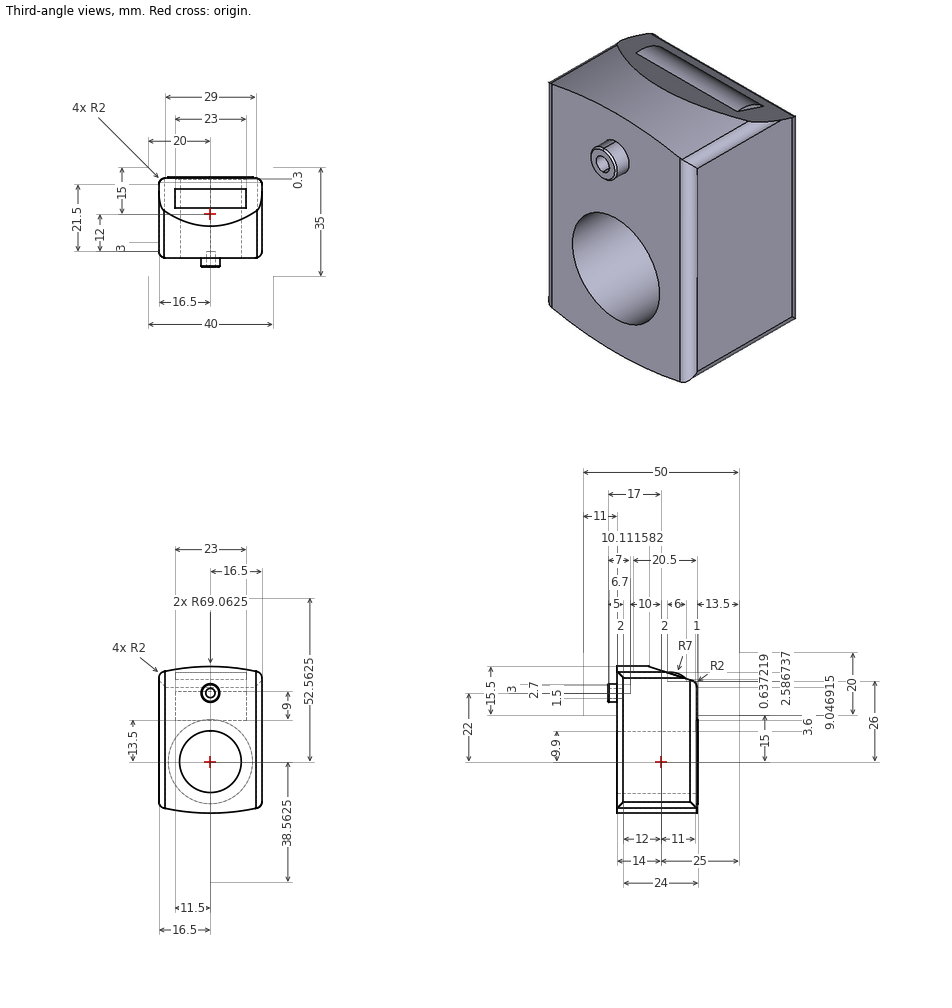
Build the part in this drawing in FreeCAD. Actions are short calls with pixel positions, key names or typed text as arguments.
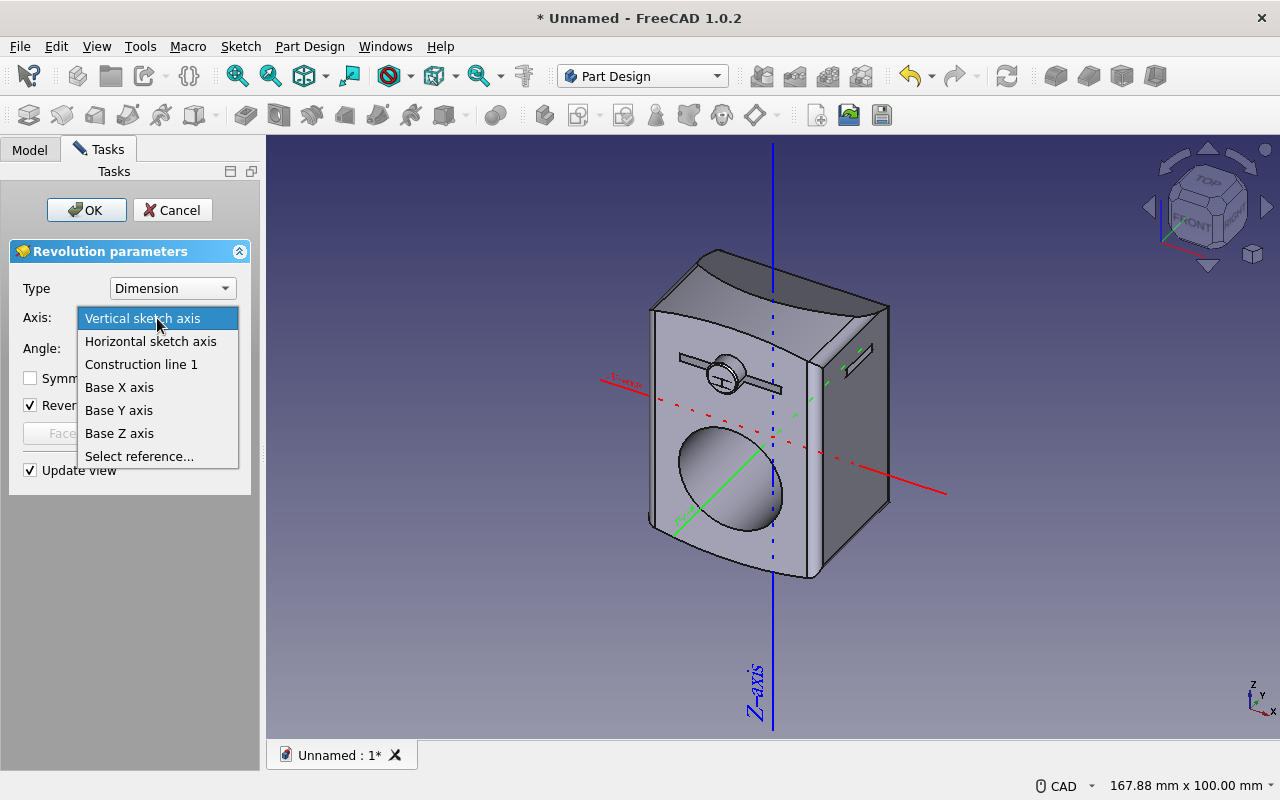
click(156, 364)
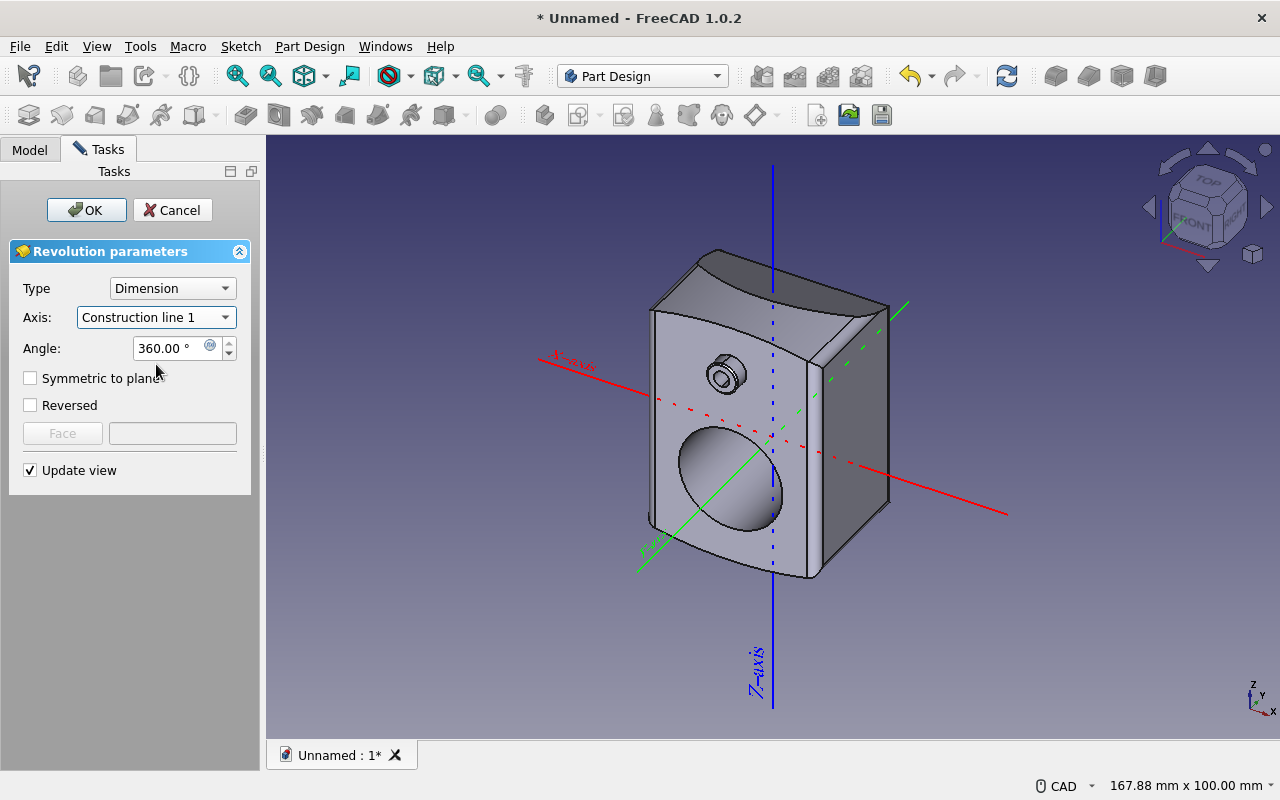
click(87, 210)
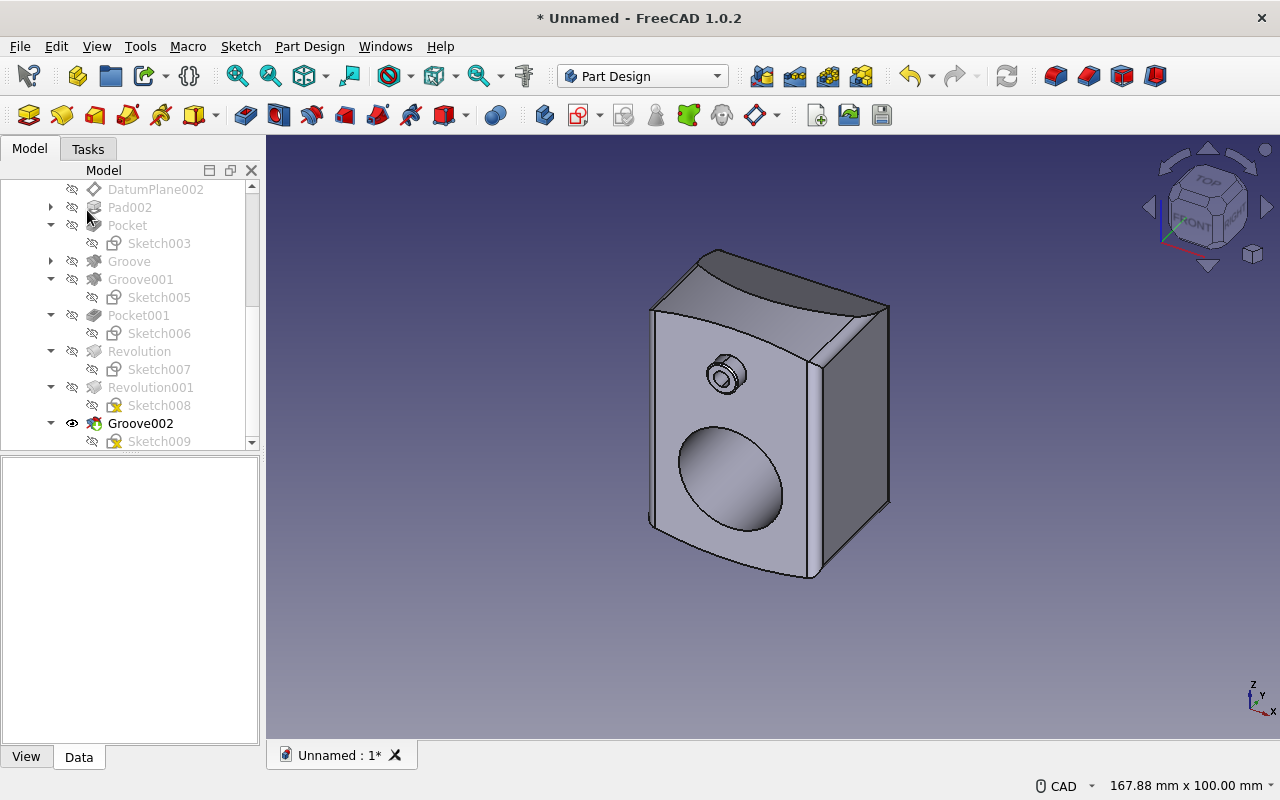
click(578, 116)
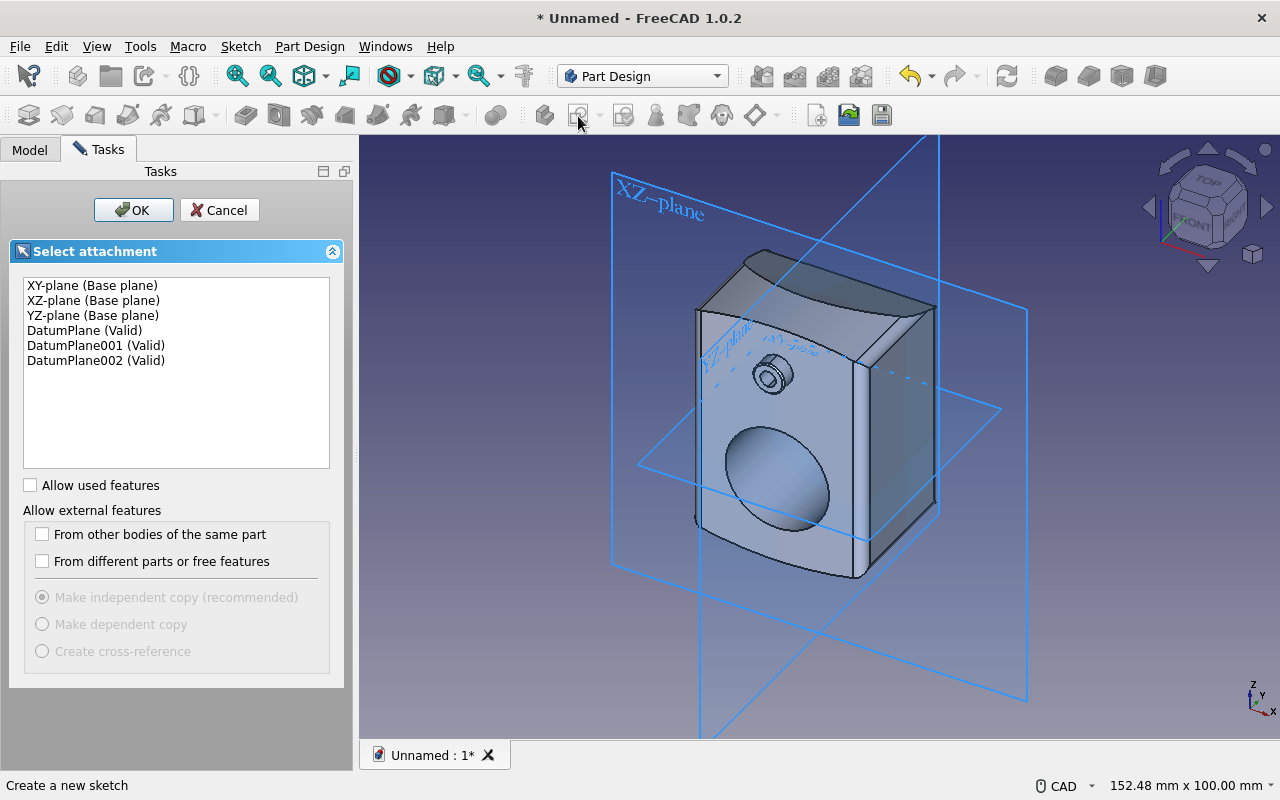
click(84, 316)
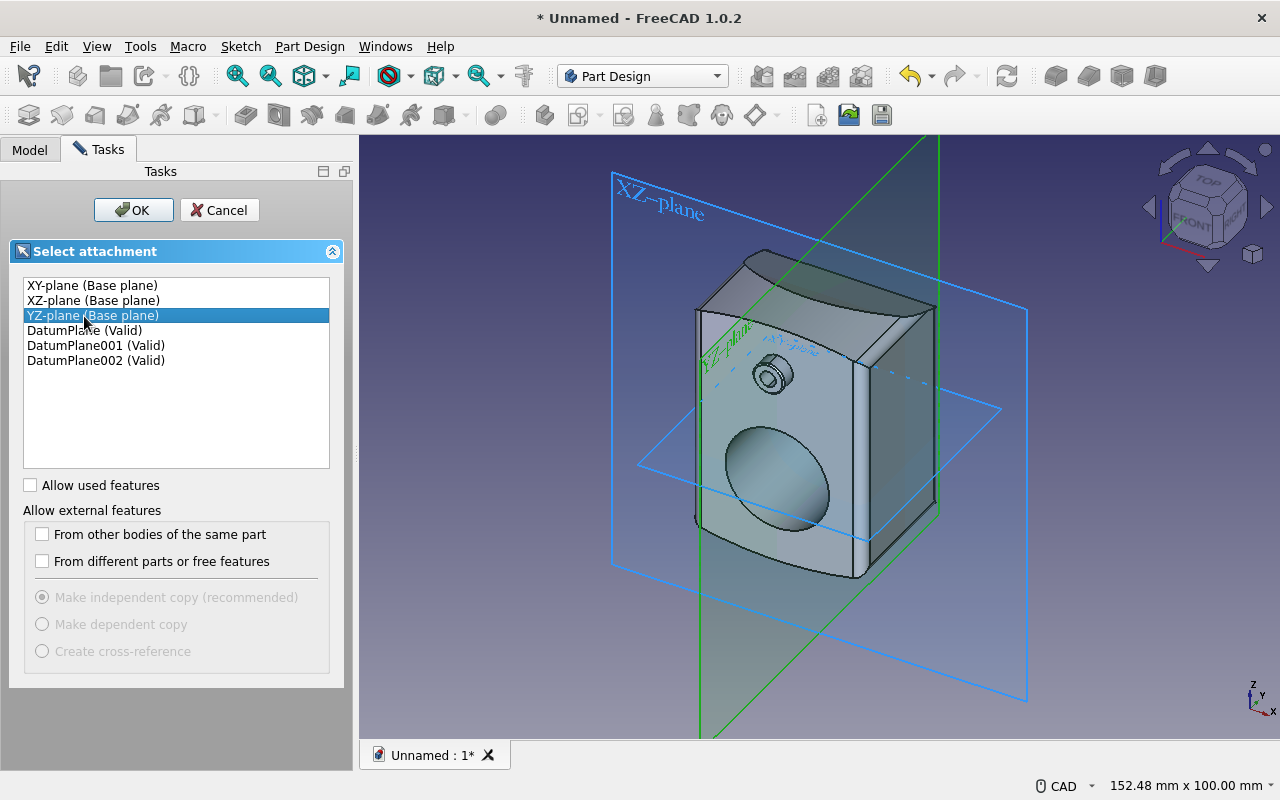
click(134, 210)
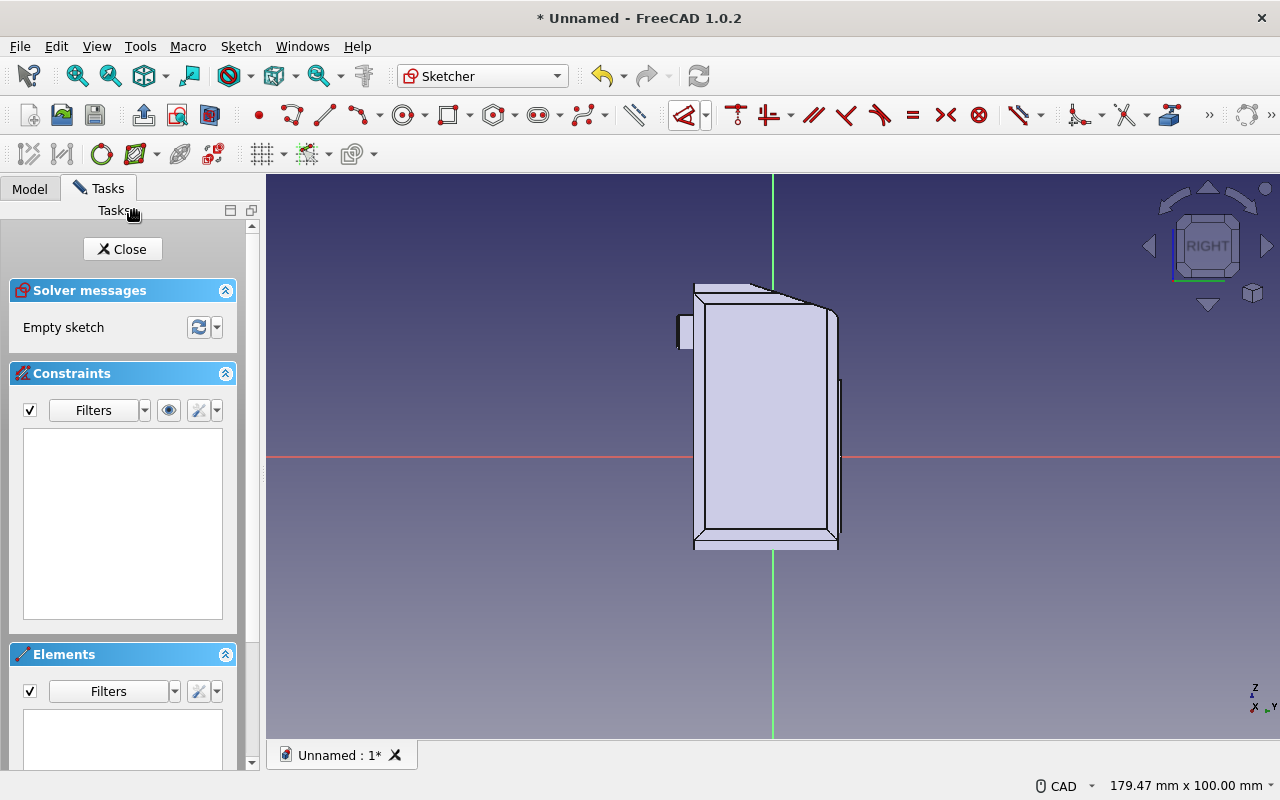
click(210, 116)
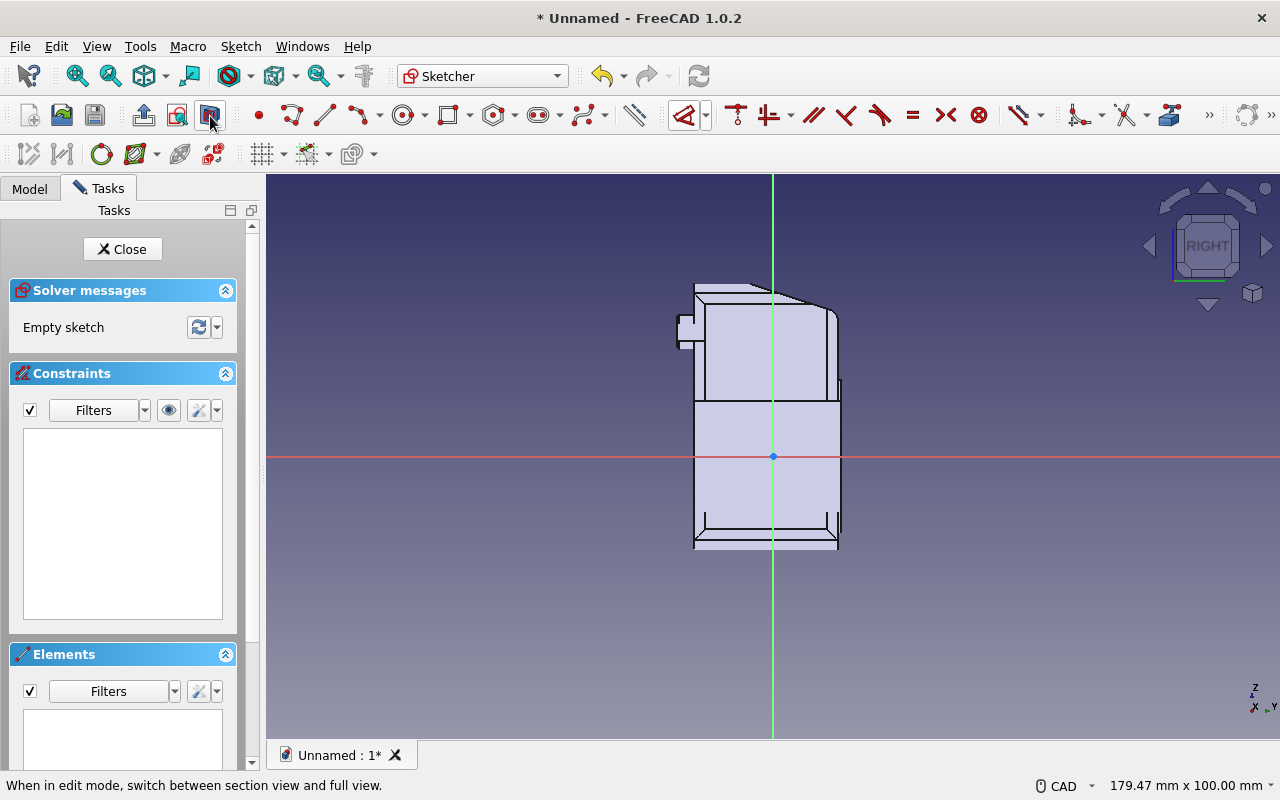
scroll(808, 292, up, 14)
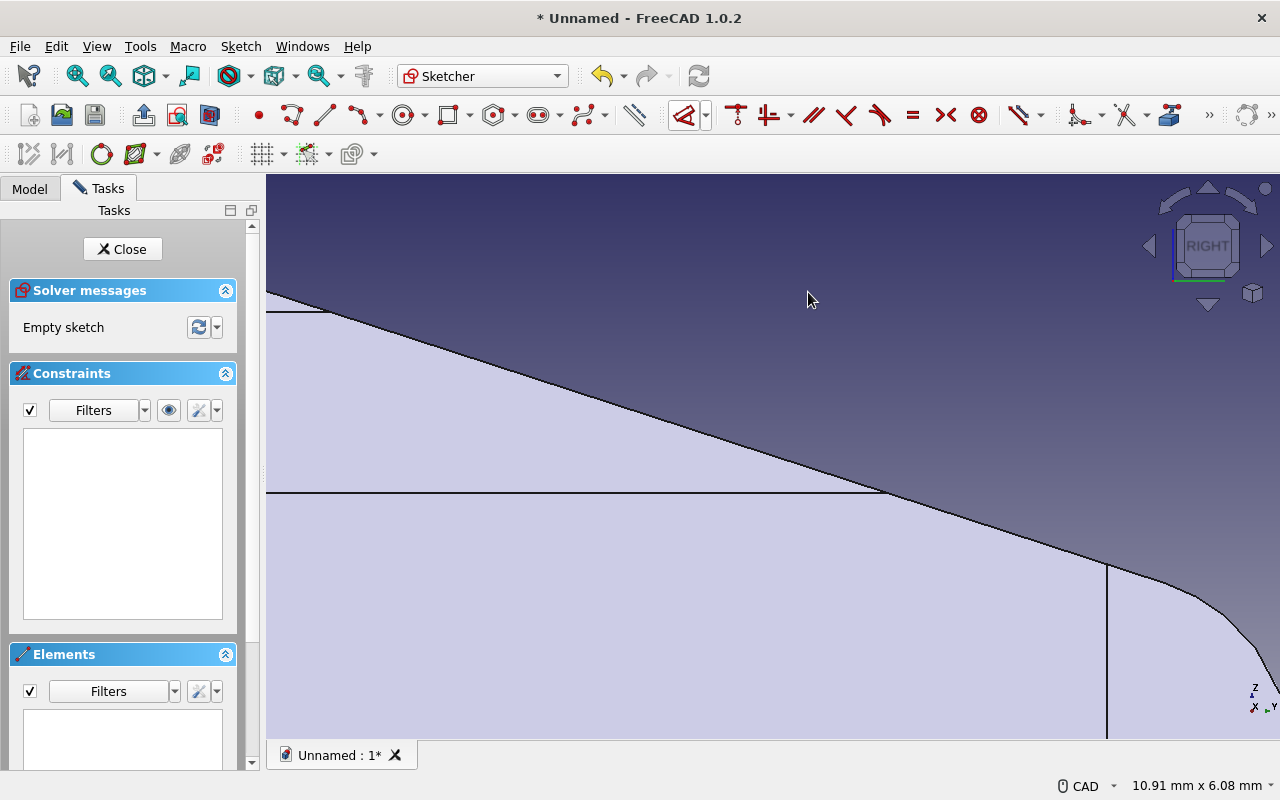
click(292, 116)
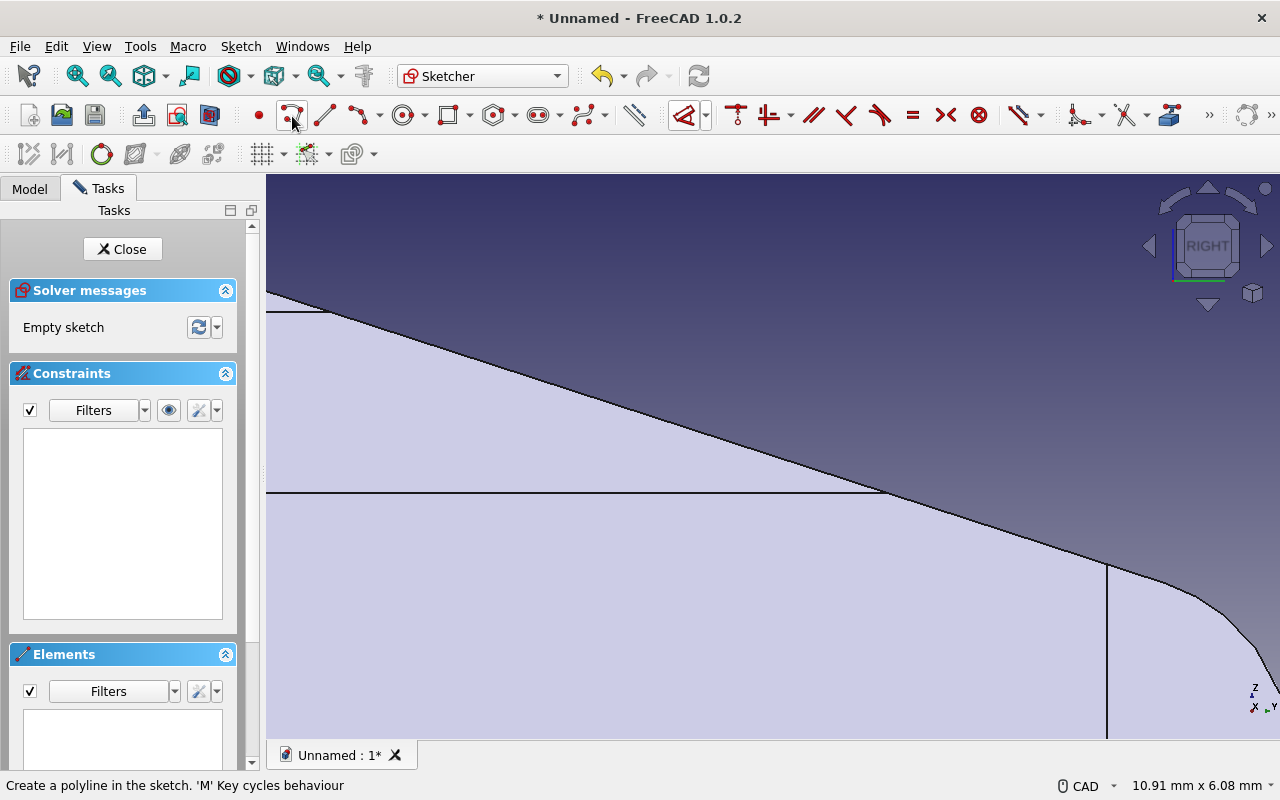
click(410, 338)
click(410, 578)
click(967, 578)
click(967, 519)
right_click(967, 519)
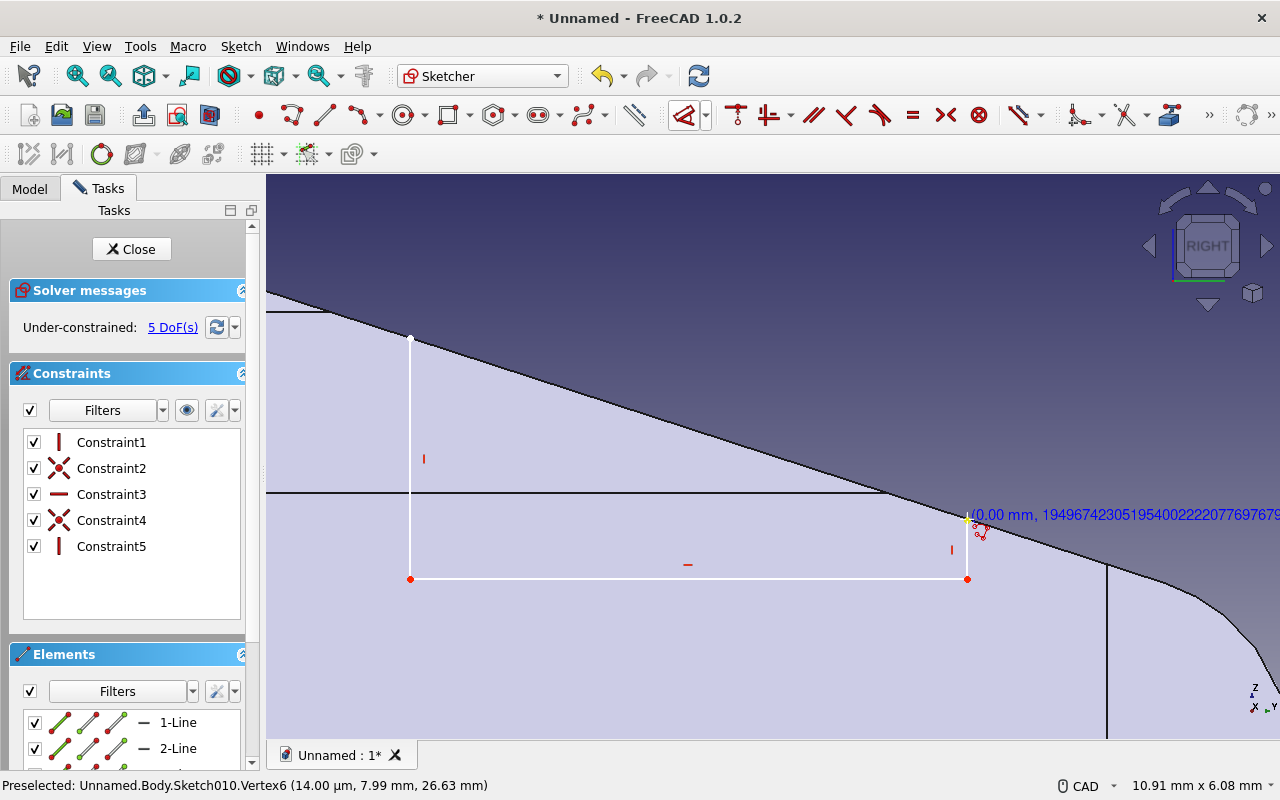
click(358, 116)